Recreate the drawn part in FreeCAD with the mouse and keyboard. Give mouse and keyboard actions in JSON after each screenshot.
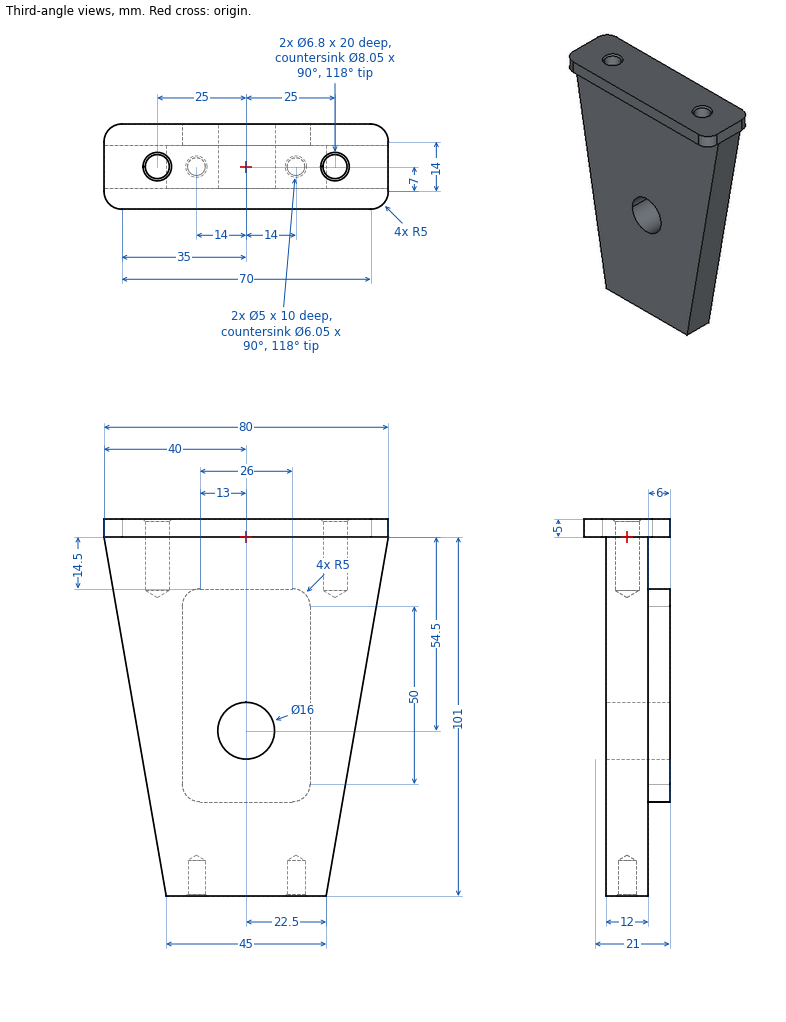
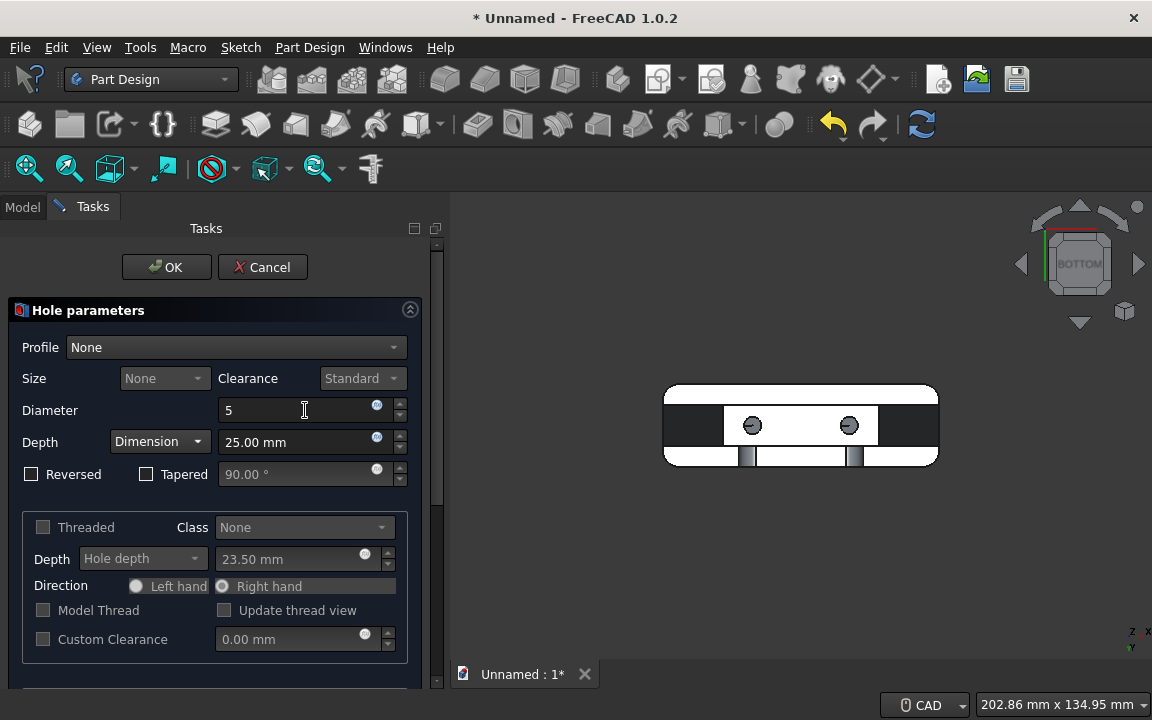
{"action": "triple_click", "coordinate": [305, 442]}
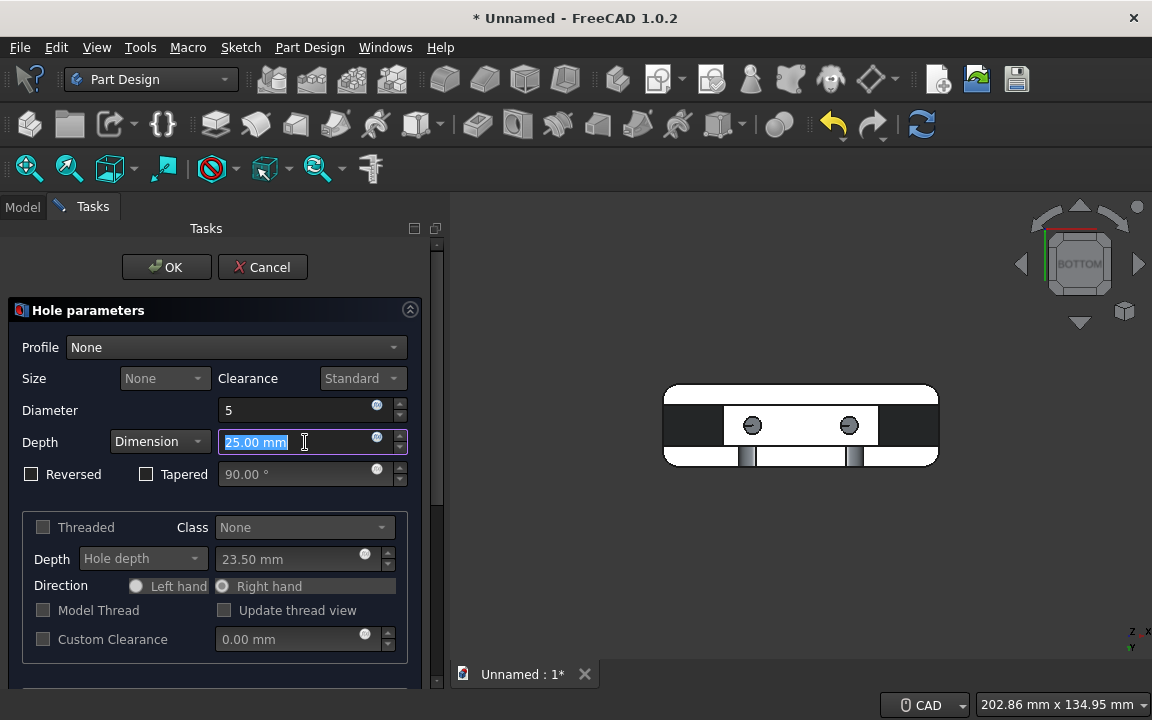
{"action": "type", "text": "10"}
{"action": "key", "text": "Tab"}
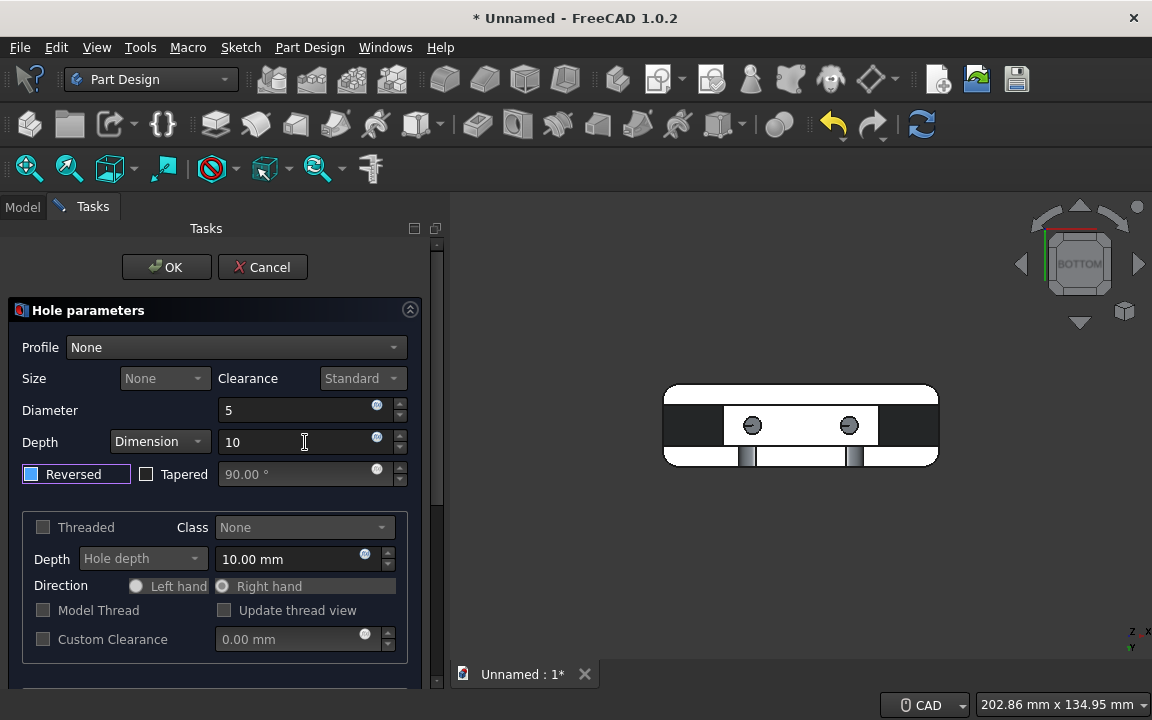
{"action": "scroll", "coordinate": [437, 463], "scroll_direction": "down", "scroll_amount": 2}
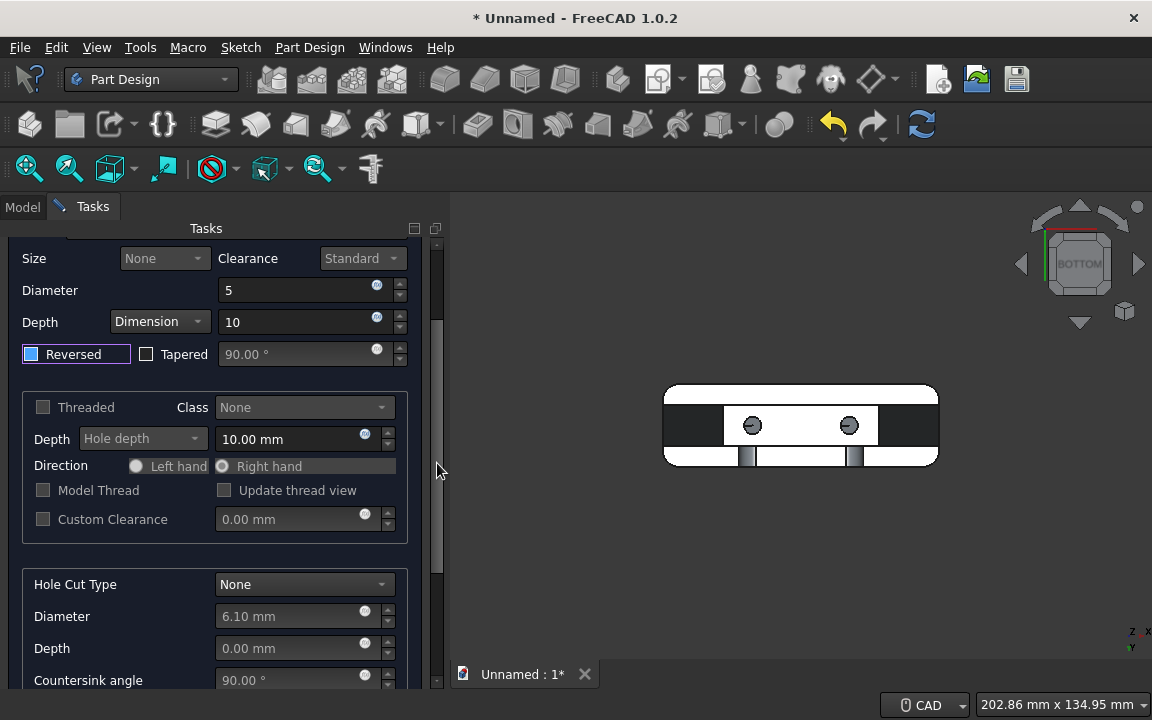
{"action": "left_click", "coordinate": [306, 584]}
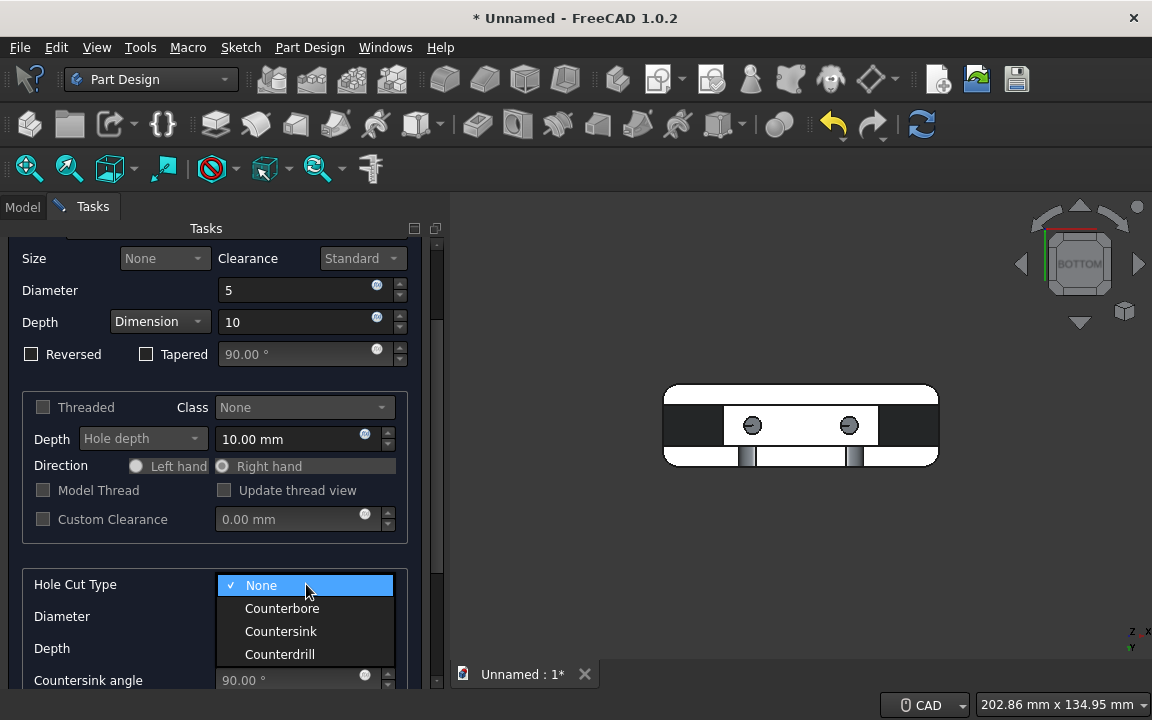
{"action": "left_click", "coordinate": [304, 632]}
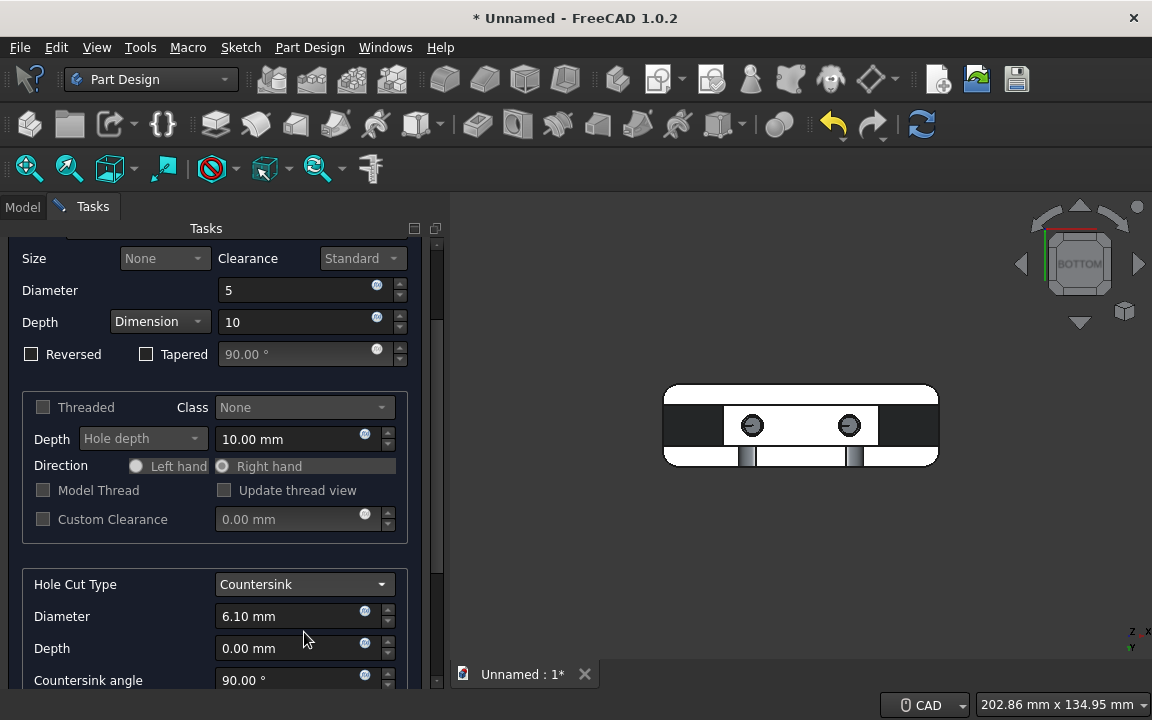
{"action": "triple_click", "coordinate": [298, 616]}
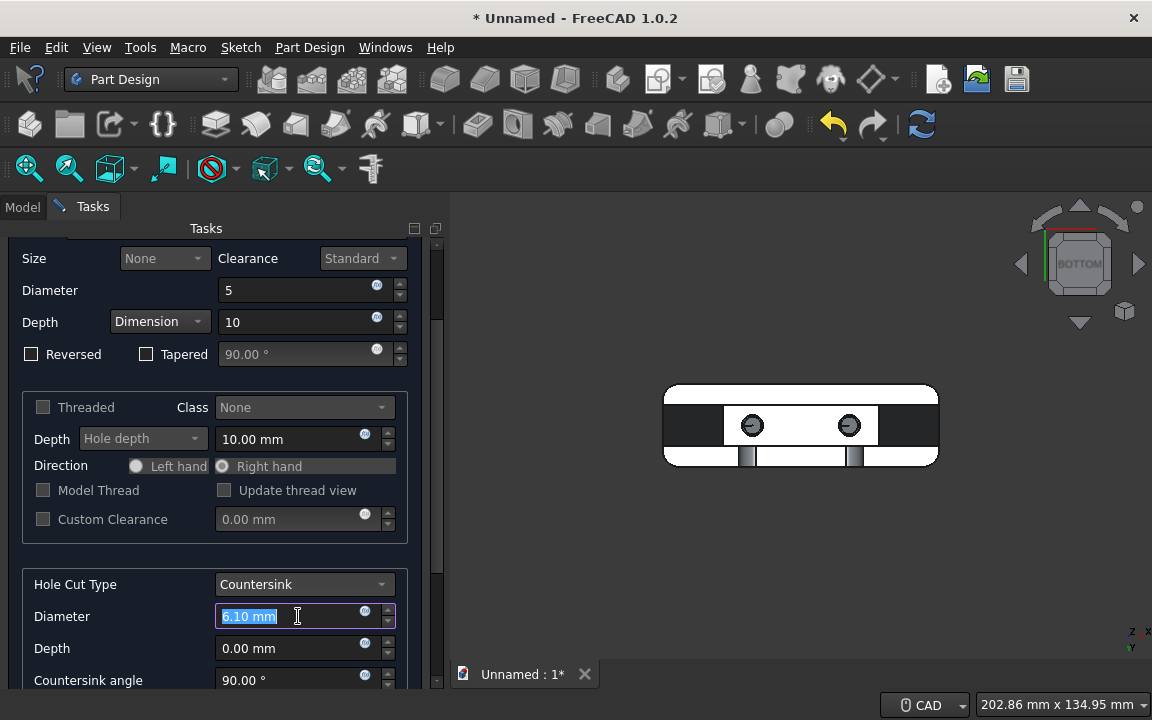
{"action": "type", "text": "6.05"}
{"action": "key", "text": "Tab"}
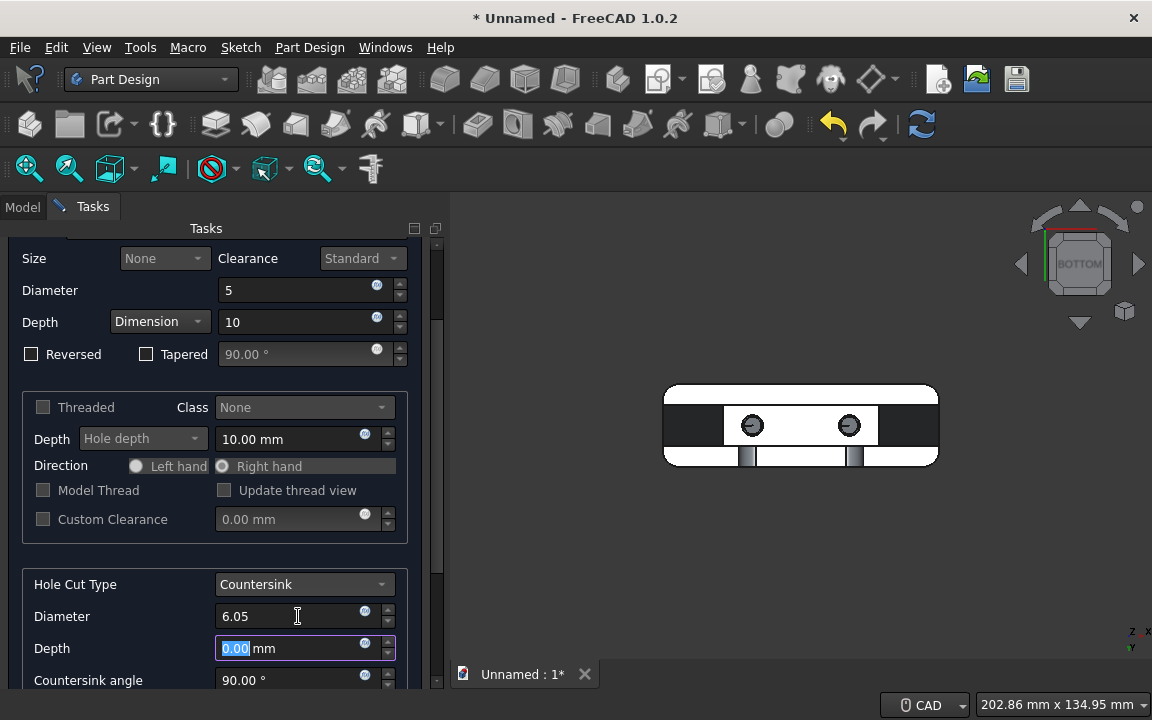
{"action": "scroll", "coordinate": [437, 463], "scroll_direction": "up", "scroll_amount": 3}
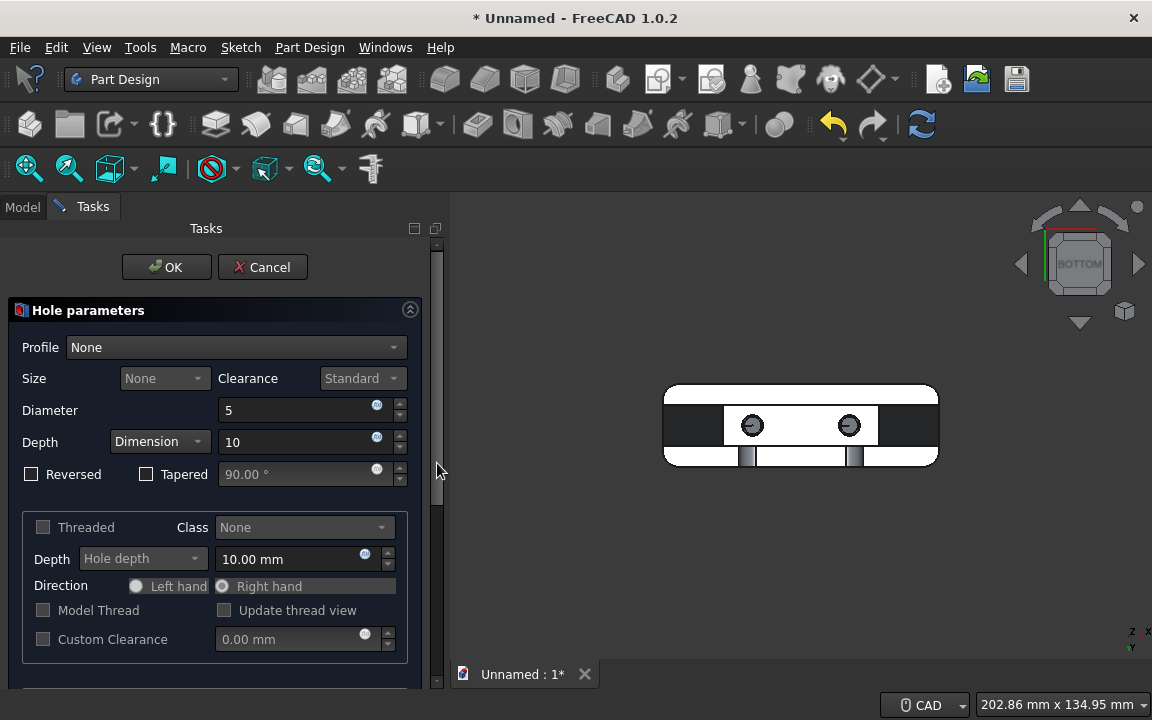
{"action": "left_click", "coordinate": [167, 267]}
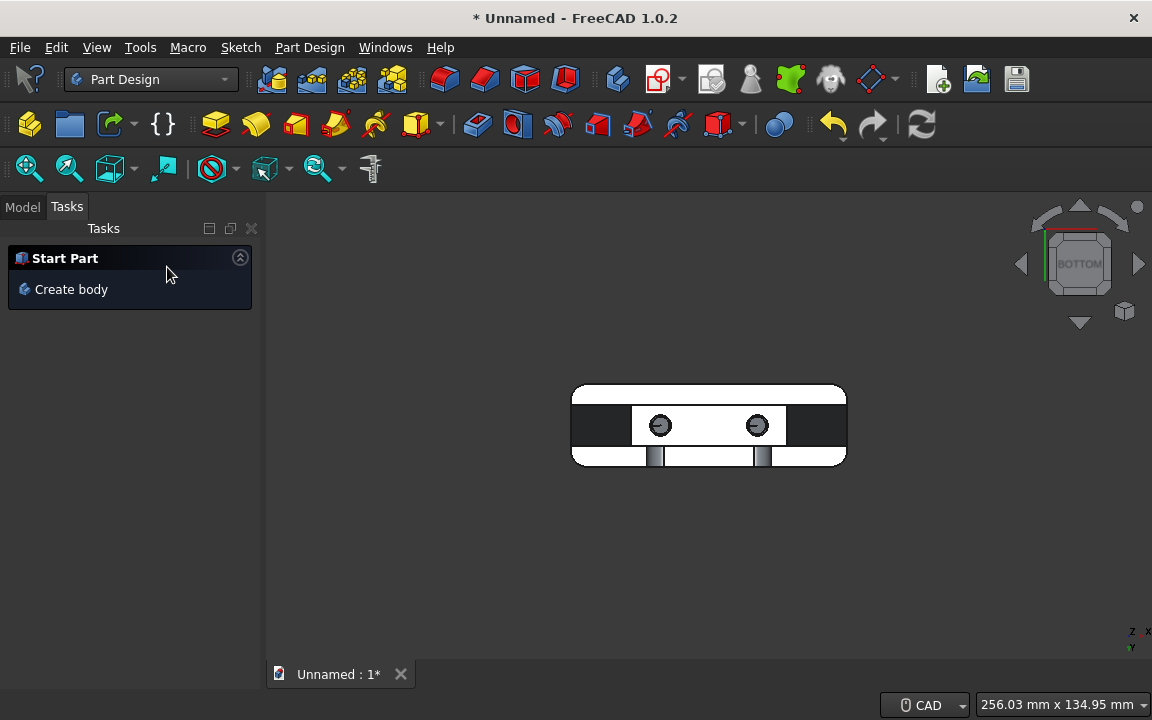
{"action": "key", "text": "0"}